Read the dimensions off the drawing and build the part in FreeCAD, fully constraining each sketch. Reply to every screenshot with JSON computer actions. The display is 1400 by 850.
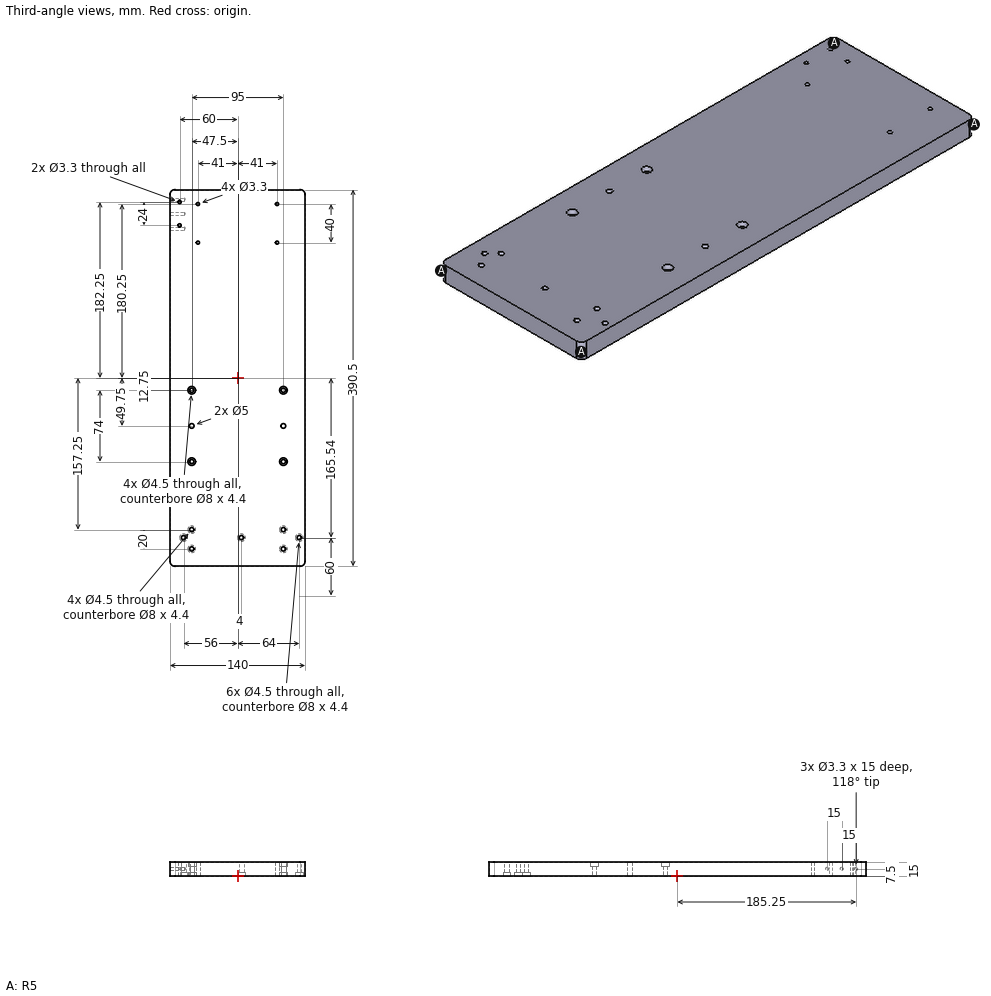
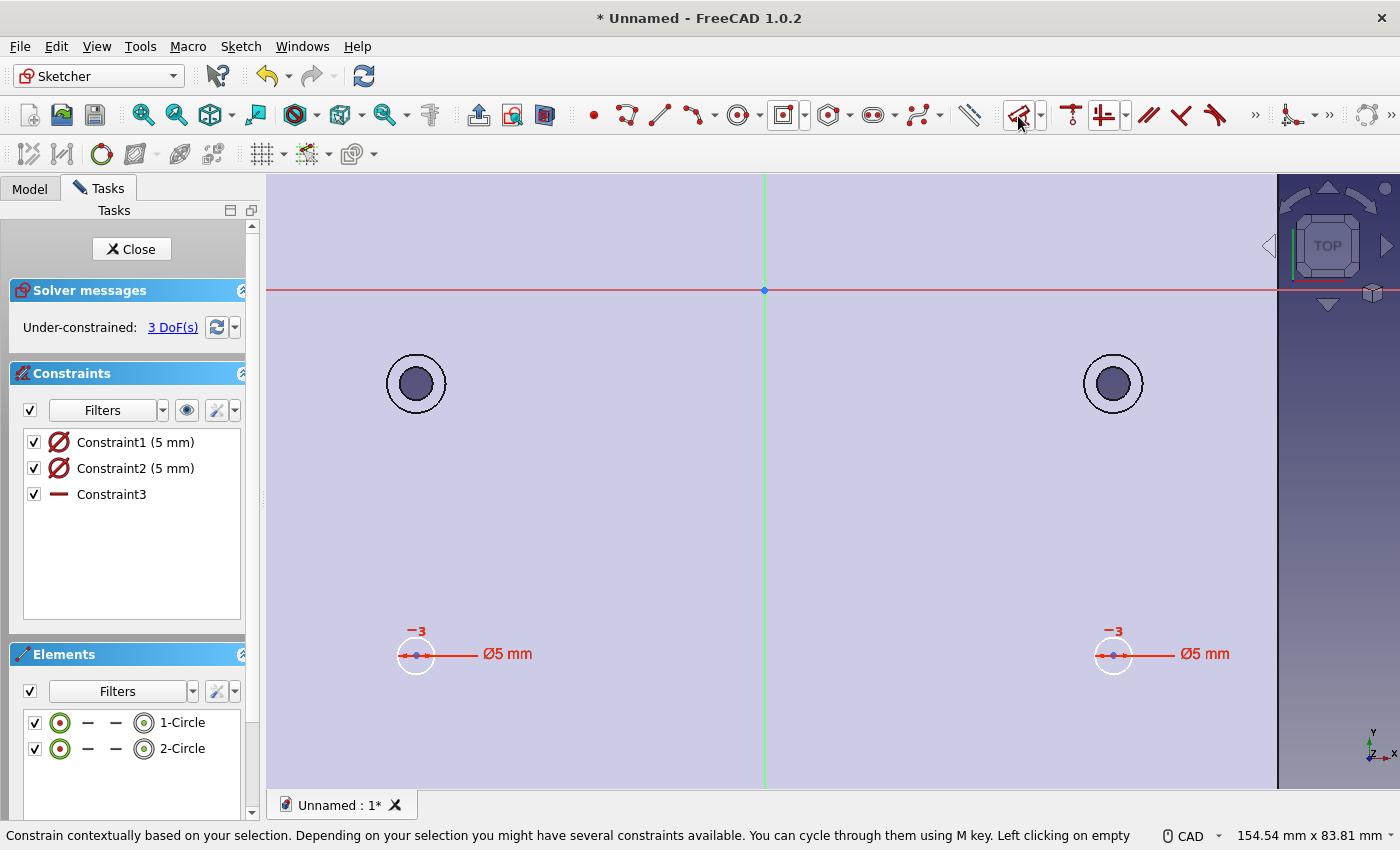
{"action": "left_click", "coordinate": [416, 656]}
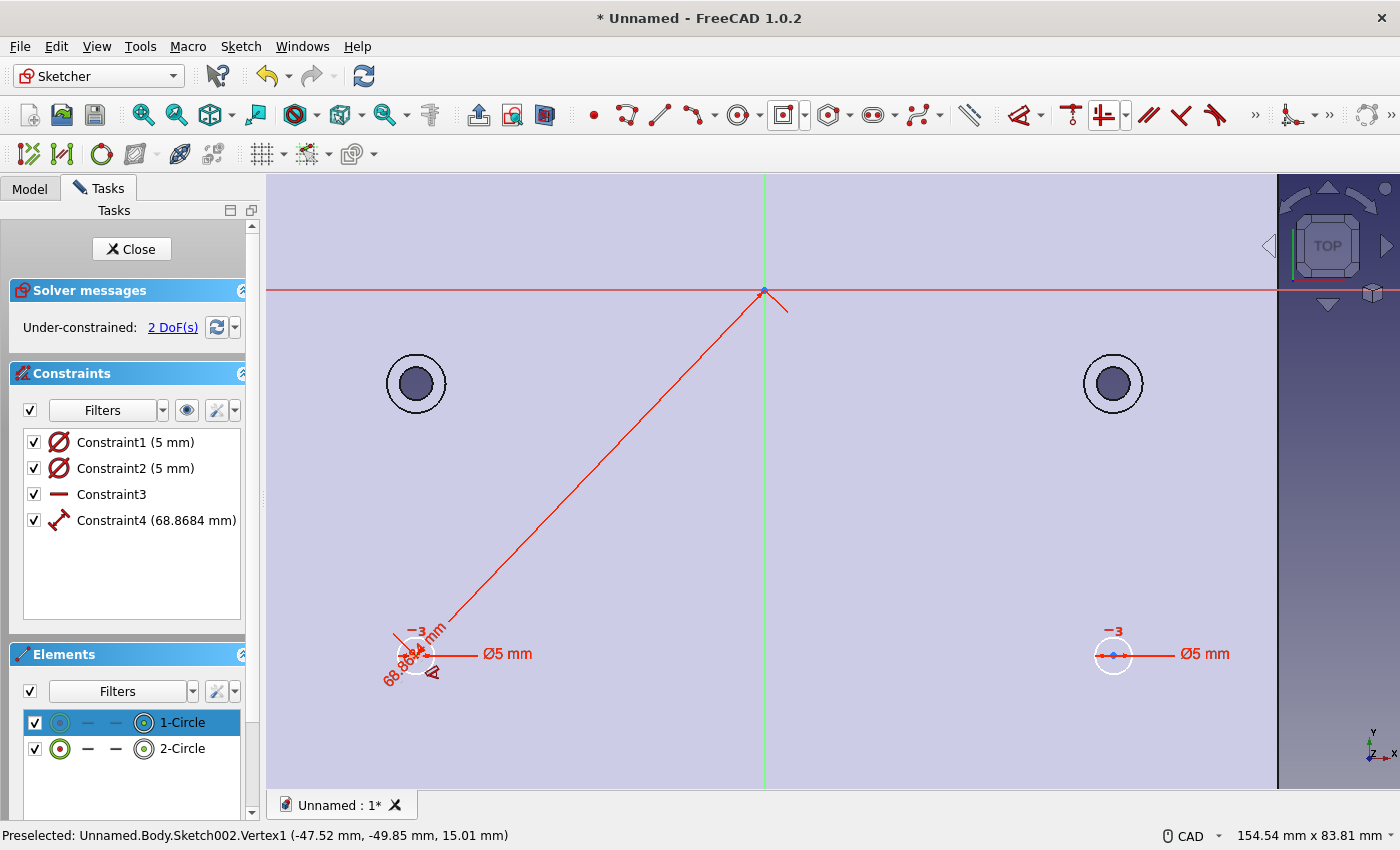
{"action": "left_click", "coordinate": [1114, 656]}
{"action": "left_click", "coordinate": [604, 690]}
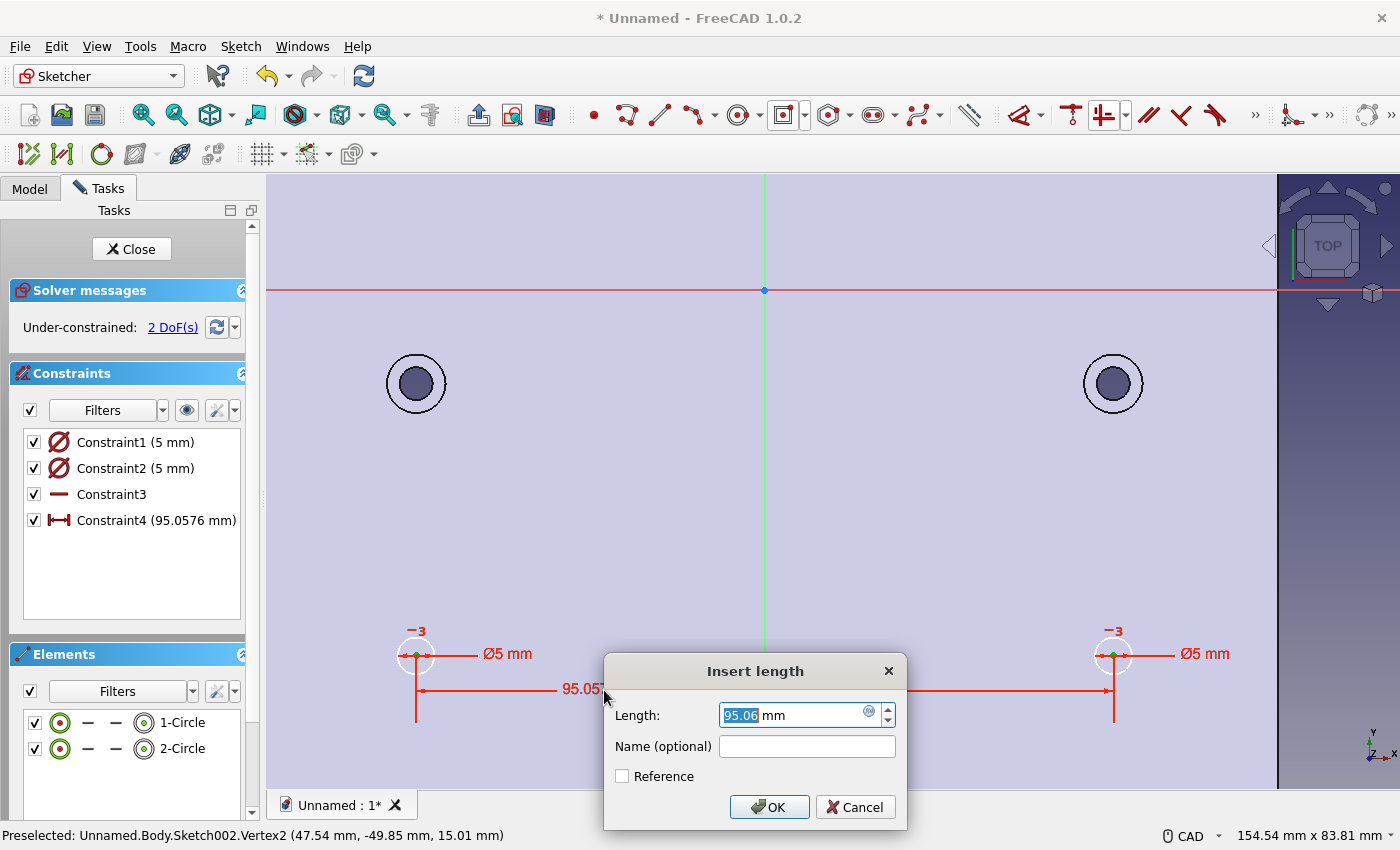
{"action": "type", "text": "95"}
{"action": "key", "text": "Return"}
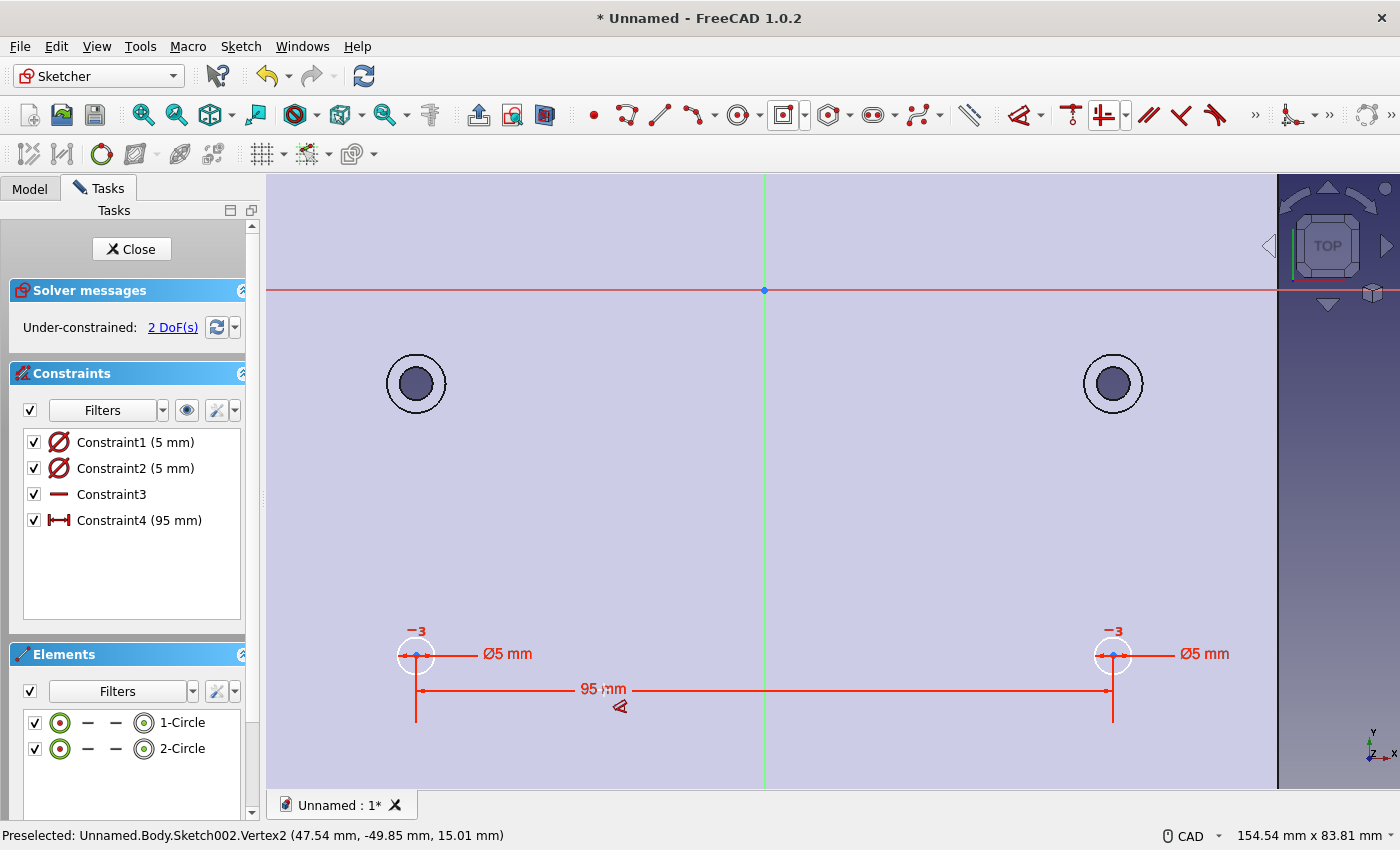
{"action": "left_click", "coordinate": [416, 656]}
{"action": "left_click", "coordinate": [590, 256]}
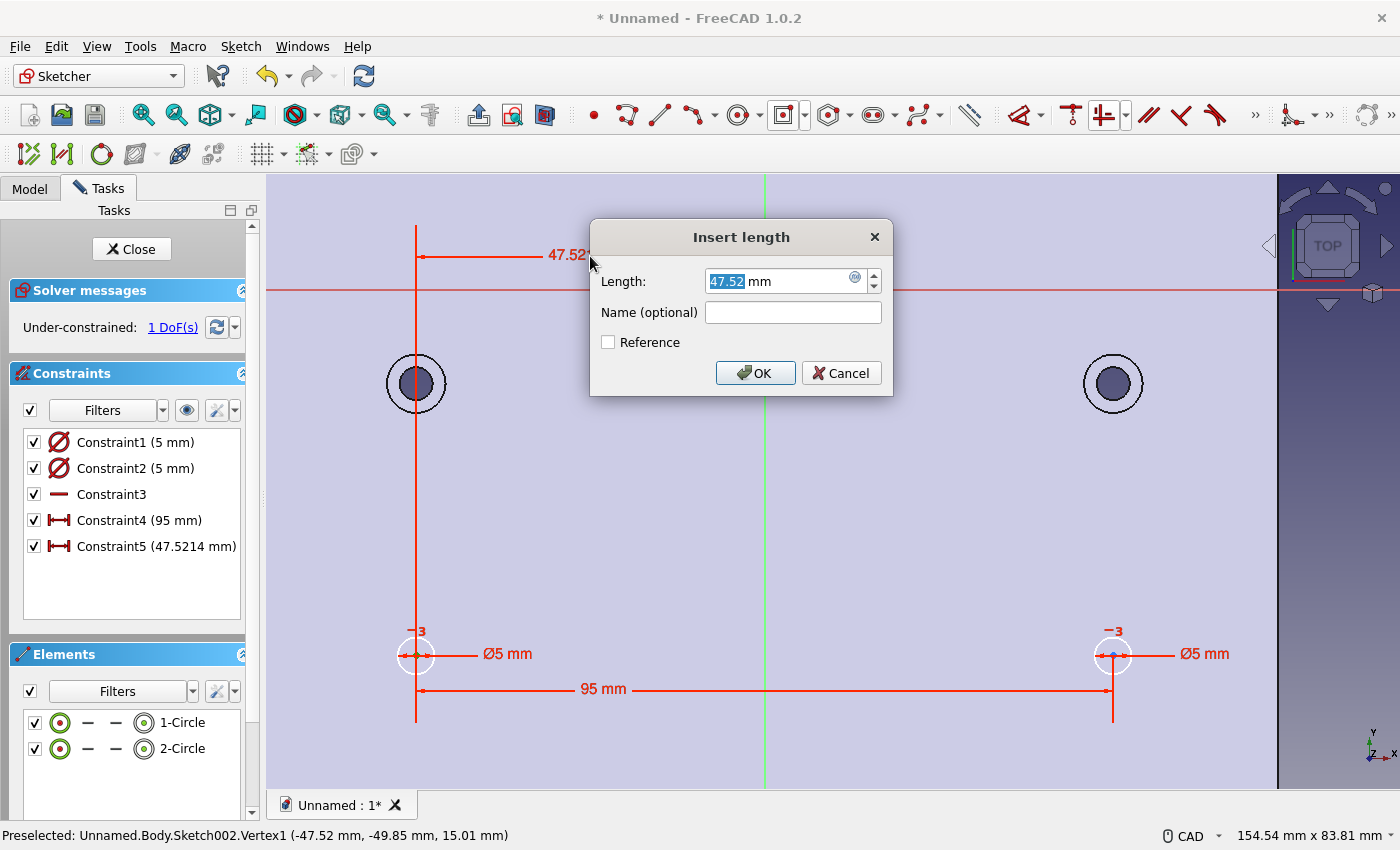
{"action": "type", "text": "47.5"}
{"action": "key", "text": "Return"}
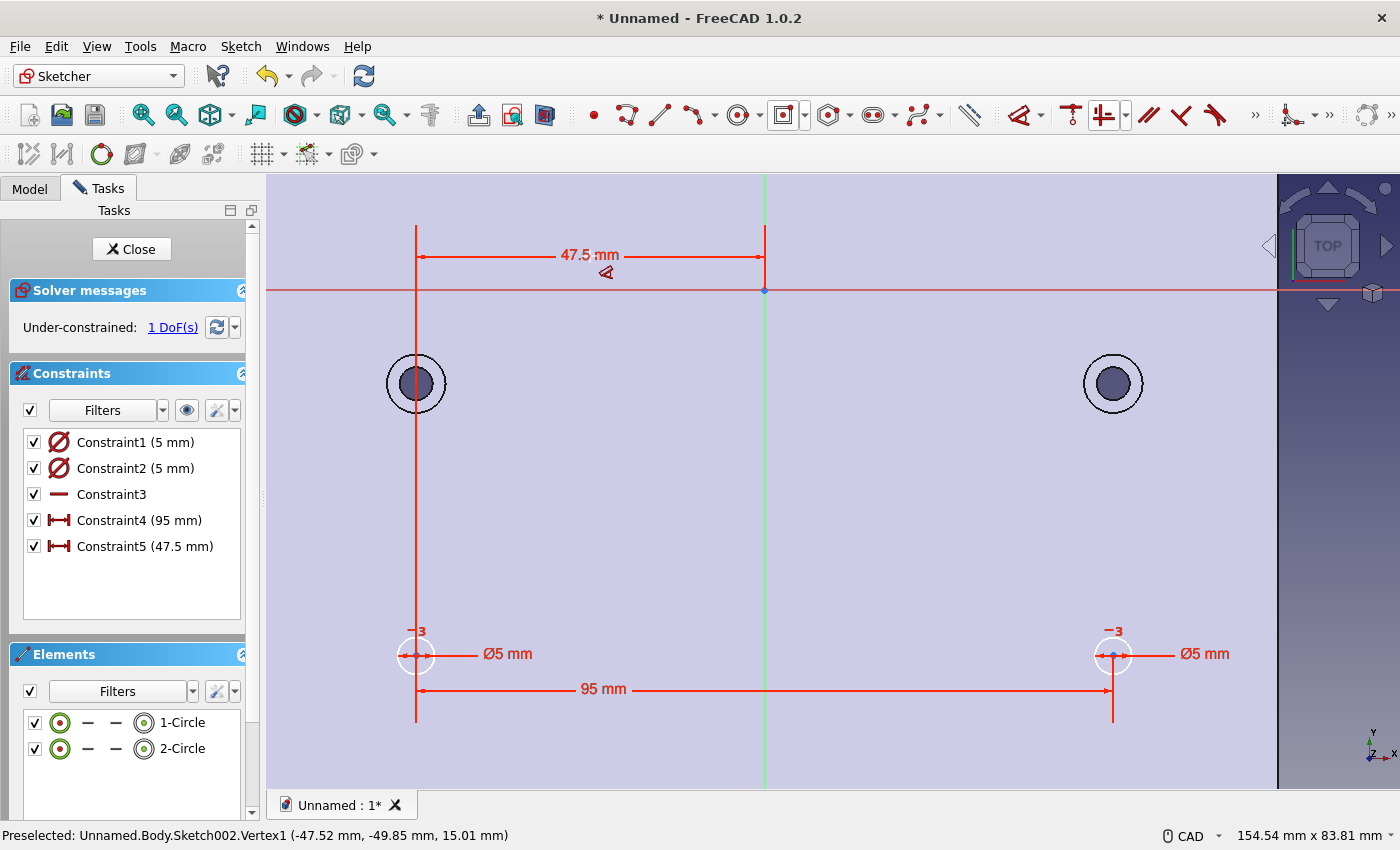
{"action": "left_click", "coordinate": [416, 656]}
{"action": "left_click", "coordinate": [382, 473]}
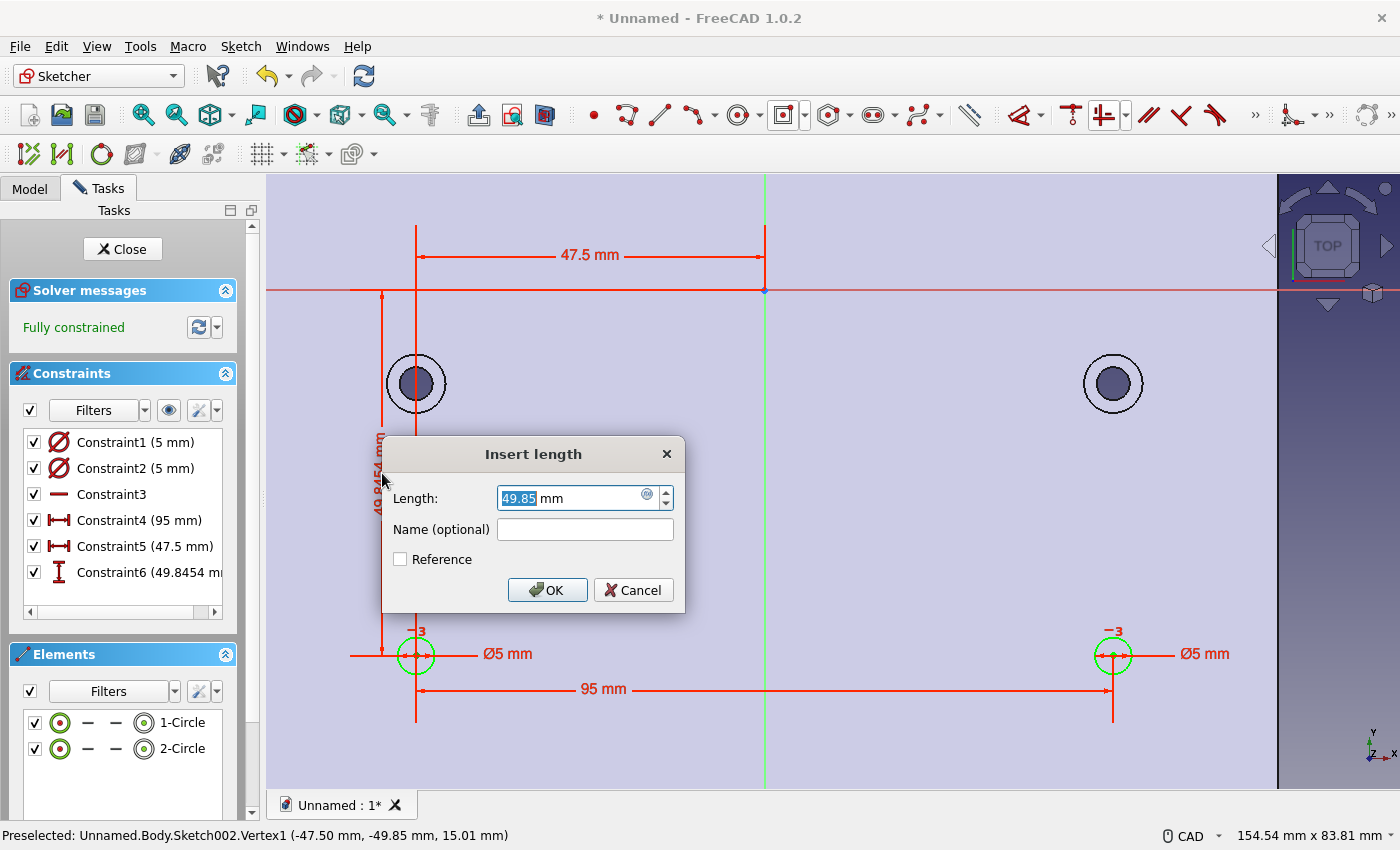
{"action": "type", "text": "49.75"}
{"action": "key", "text": "Return"}
{"action": "key", "text": "Escape"}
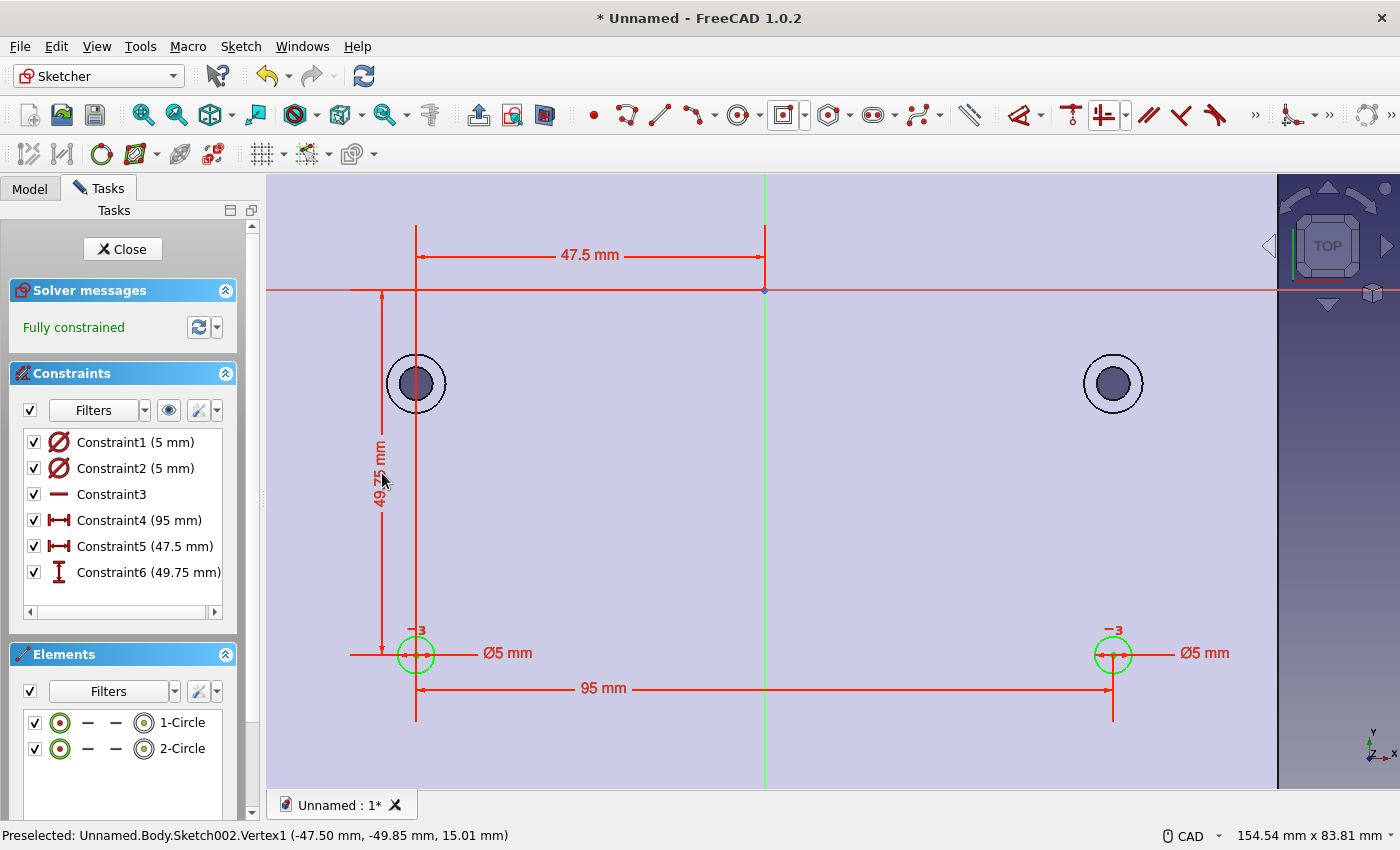
{"action": "left_click", "coordinate": [123, 249]}